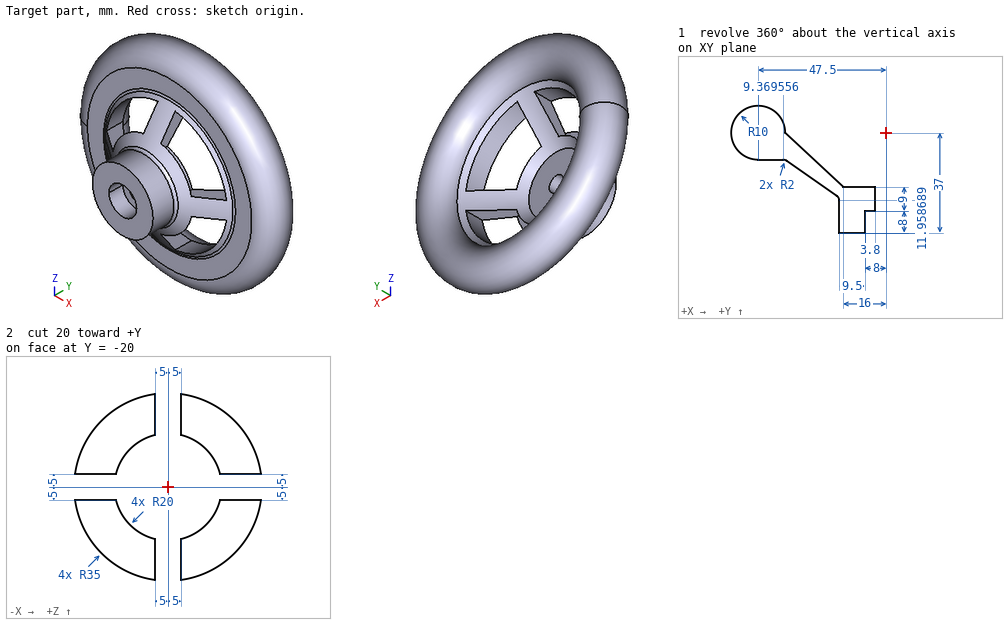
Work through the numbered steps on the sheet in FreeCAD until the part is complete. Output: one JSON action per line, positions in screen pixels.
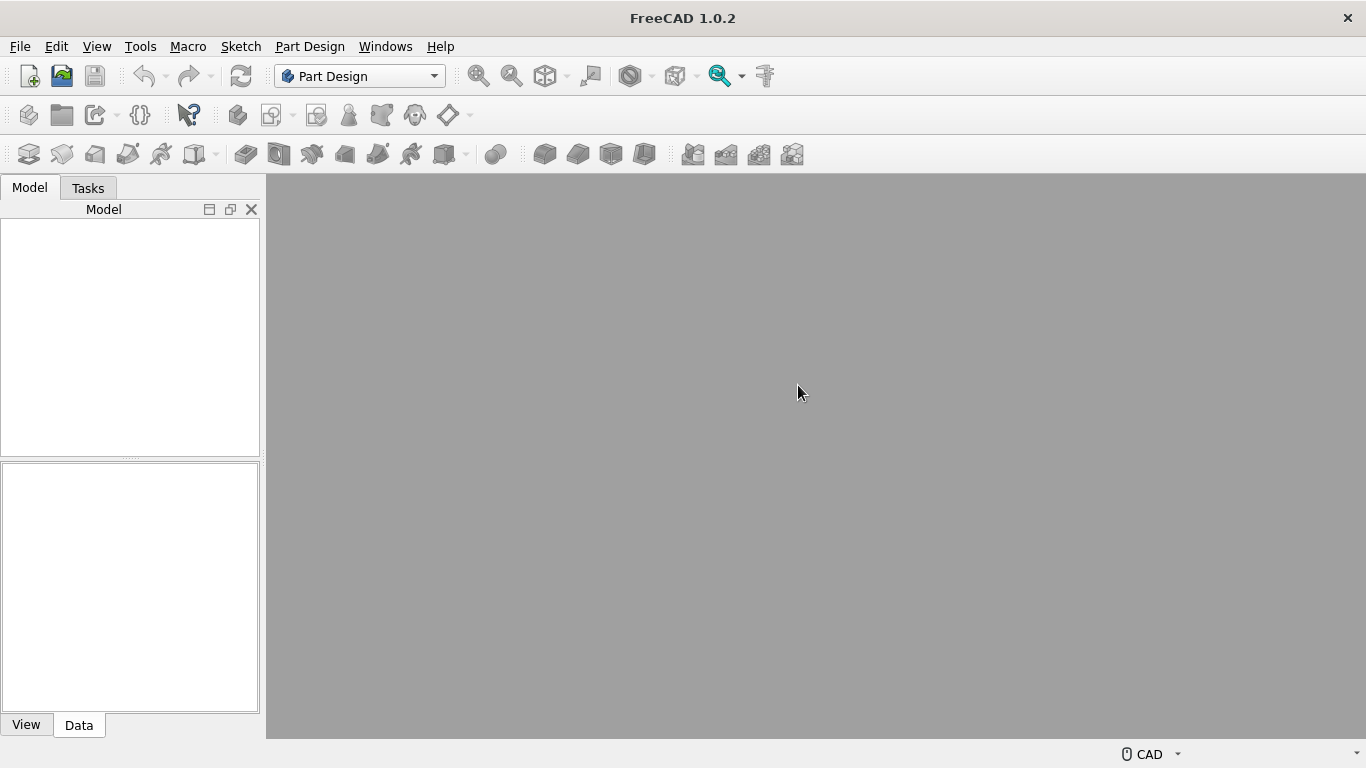
{"action": "left_click", "coordinate": [29, 76]}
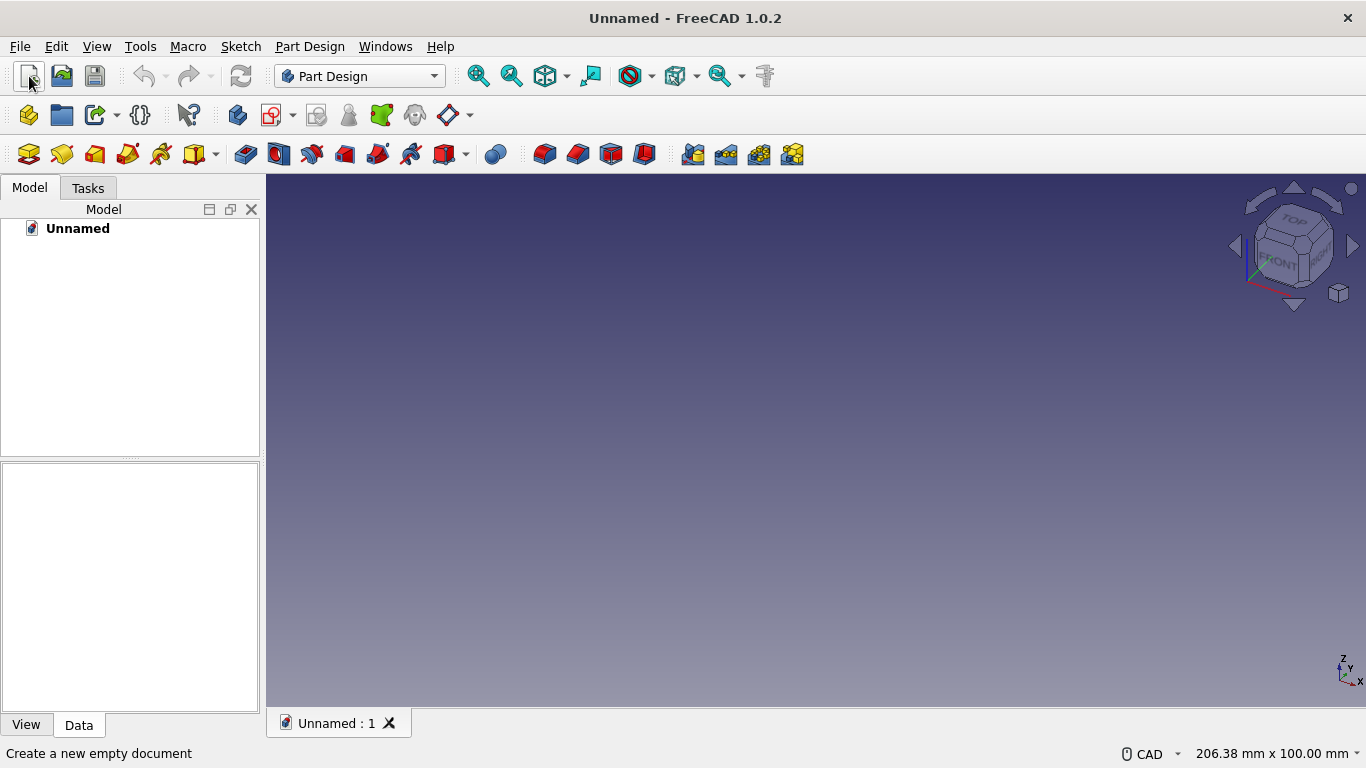
{"action": "left_click", "coordinate": [270, 116]}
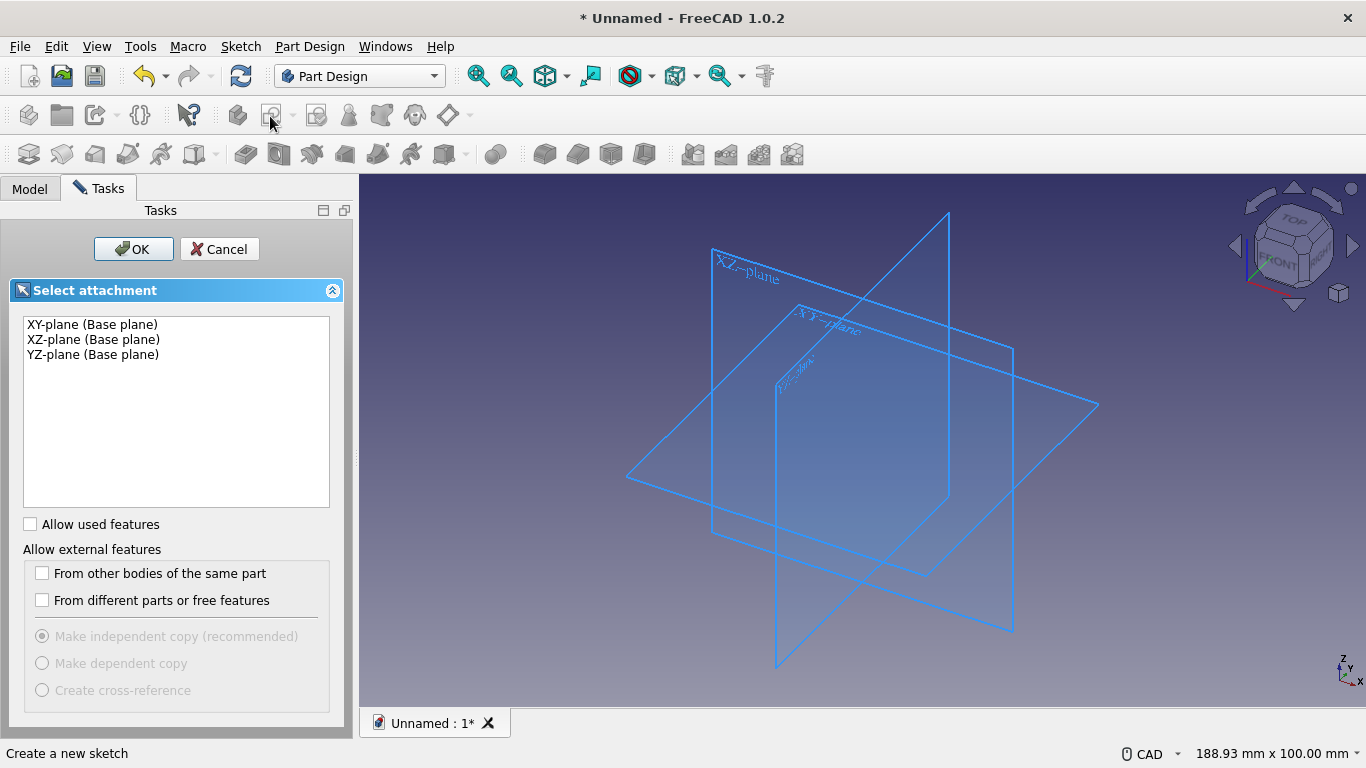
{"action": "left_click", "coordinate": [84, 324]}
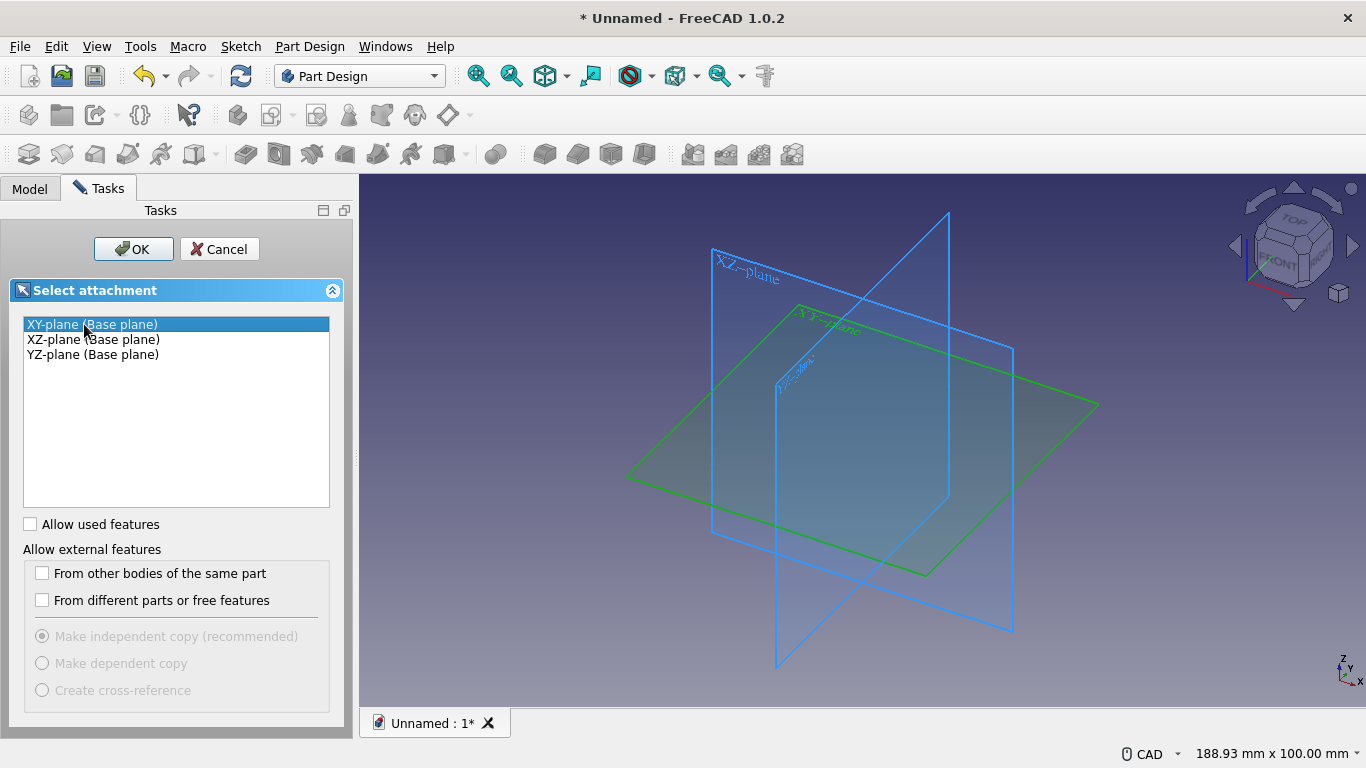
{"action": "left_click", "coordinate": [134, 249]}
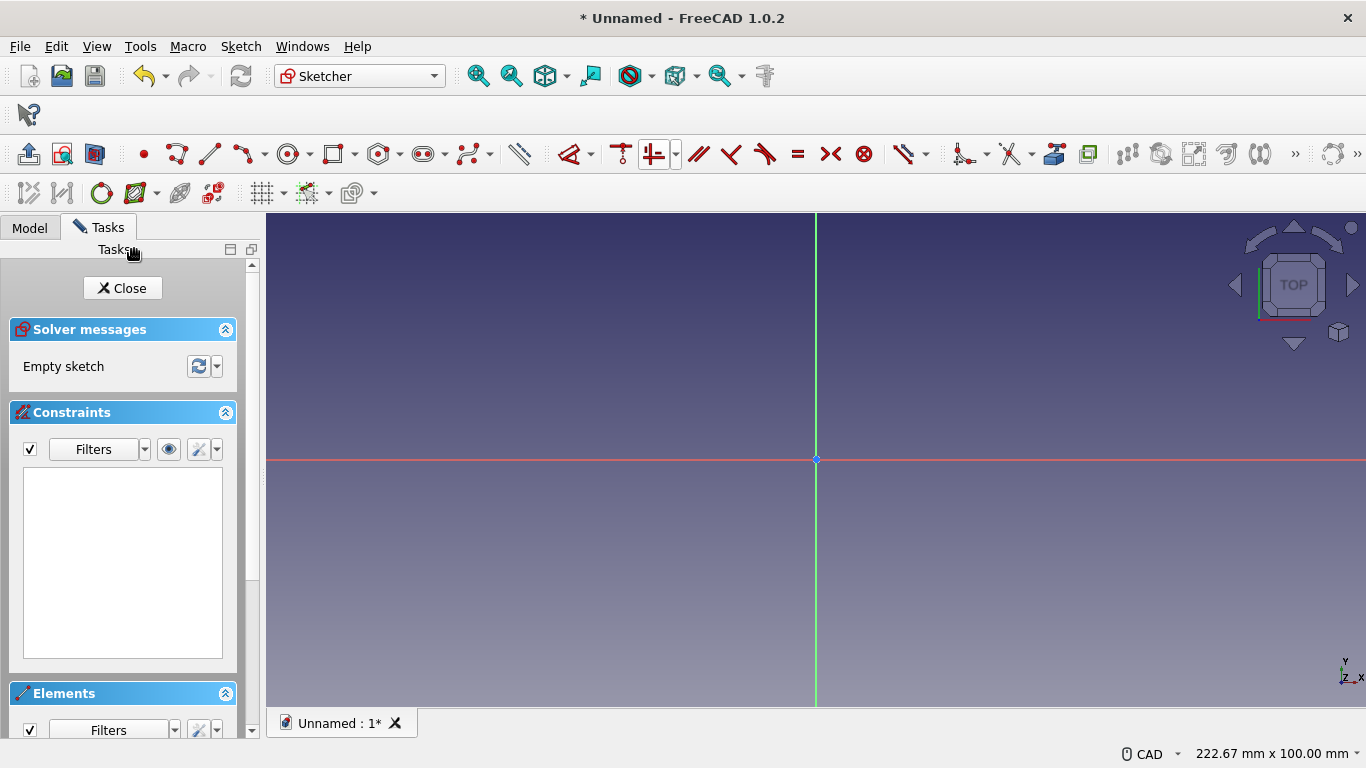
{"action": "scroll", "coordinate": [546, 679], "scroll_direction": "up", "scroll_amount": 2}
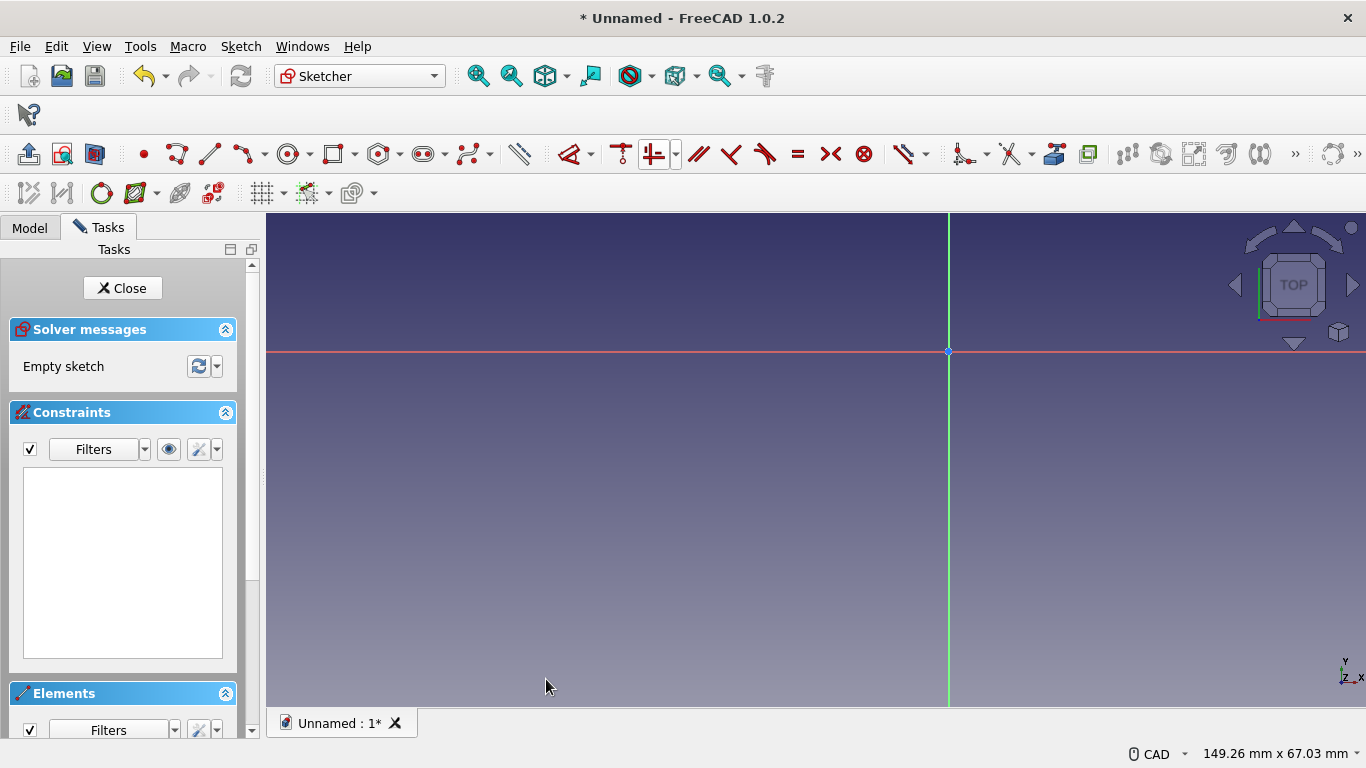
{"action": "key", "text": "g l"}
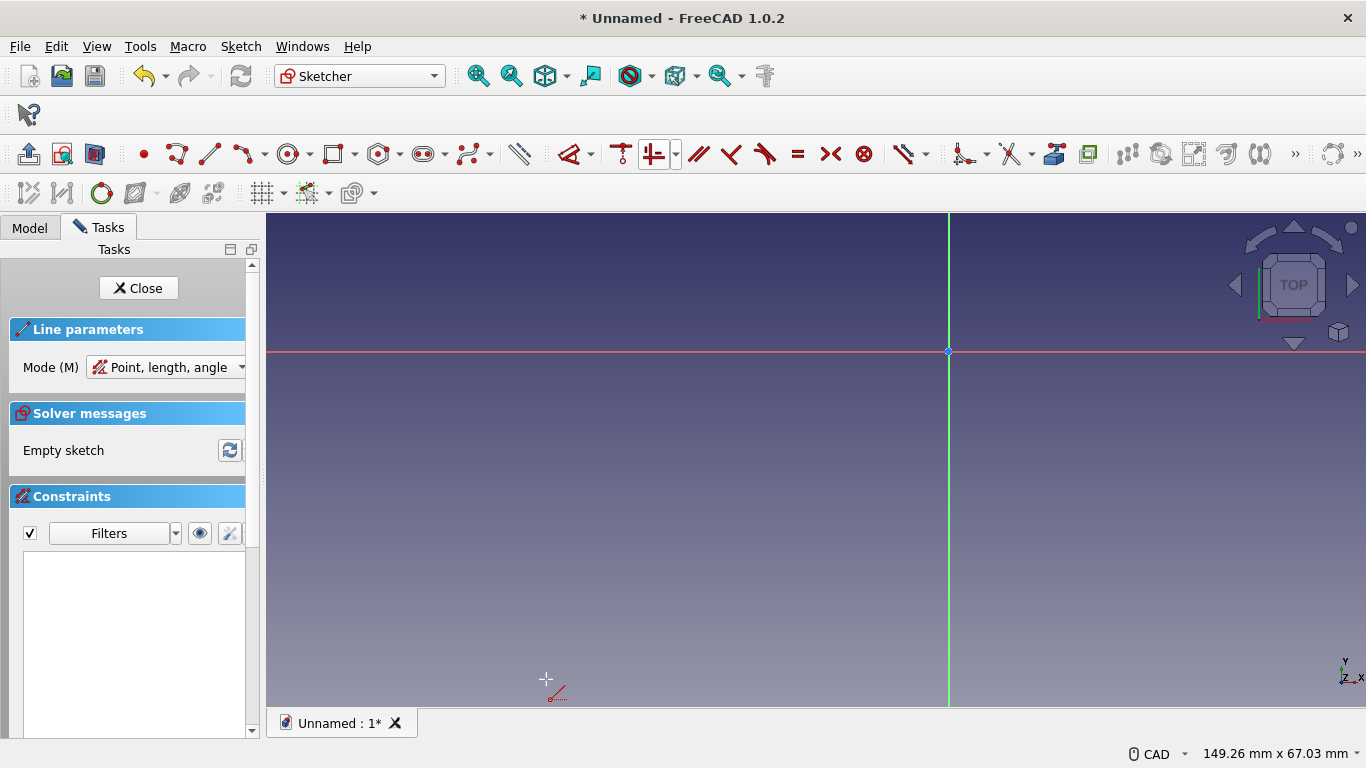
{"action": "left_click", "coordinate": [599, 426]}
{"action": "left_click", "coordinate": [668, 426]}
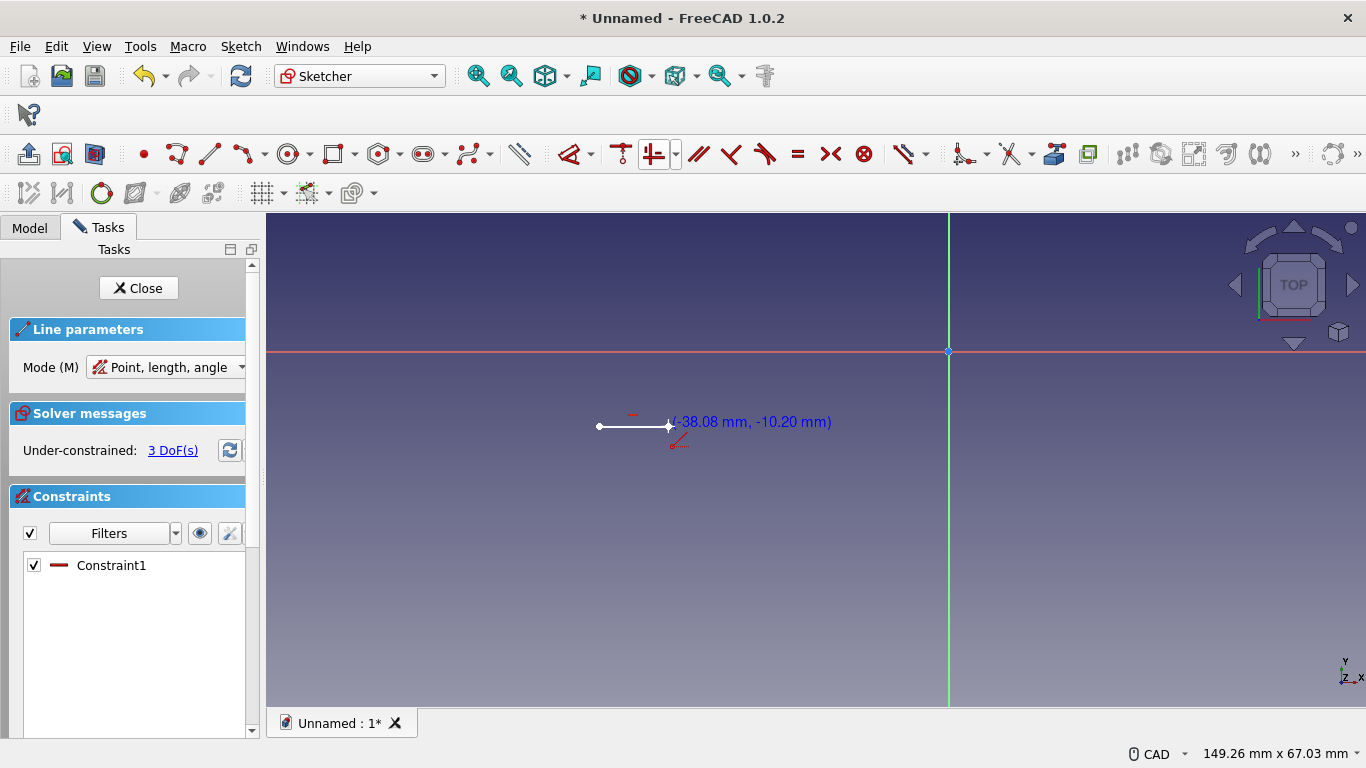
{"action": "scroll", "coordinate": [676, 428], "scroll_direction": "up", "scroll_amount": 3}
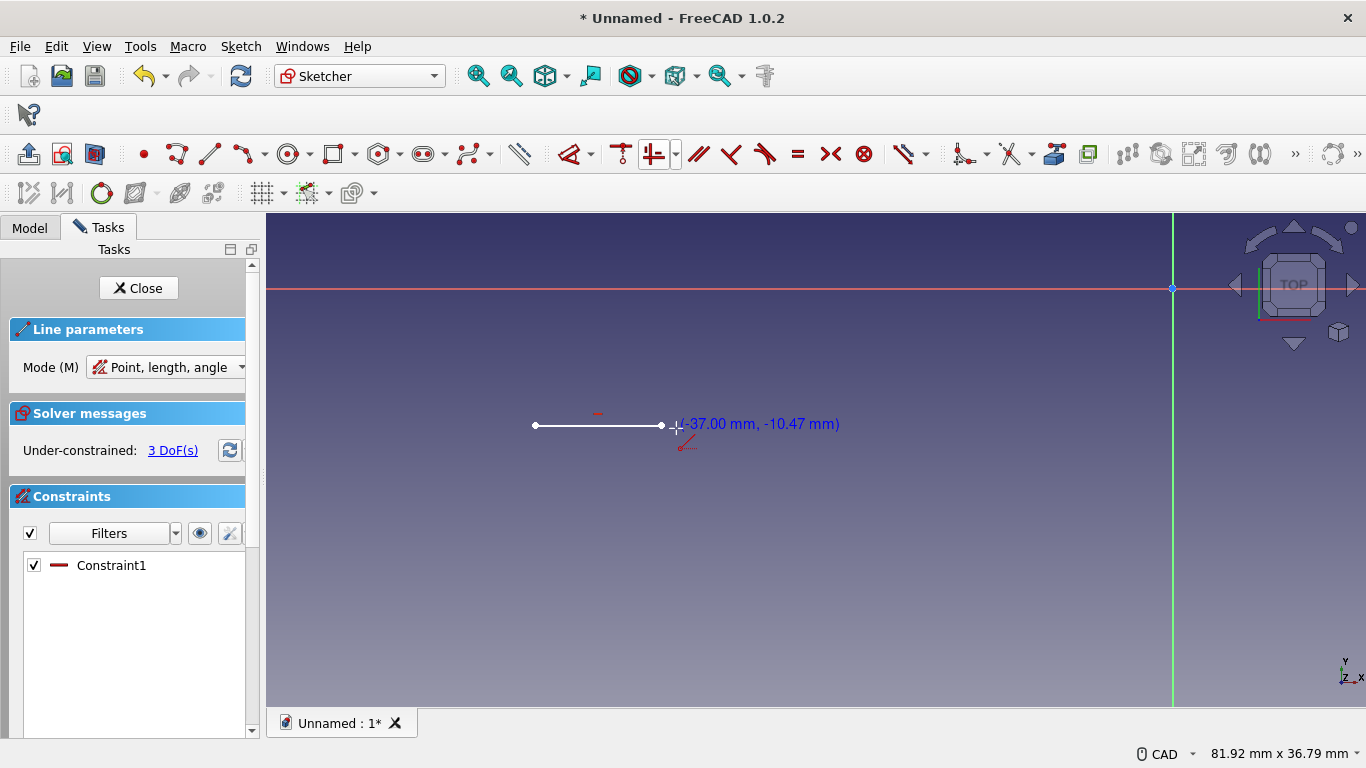
{"action": "left_click", "coordinate": [676, 428]}
{"action": "left_click", "coordinate": [926, 603]}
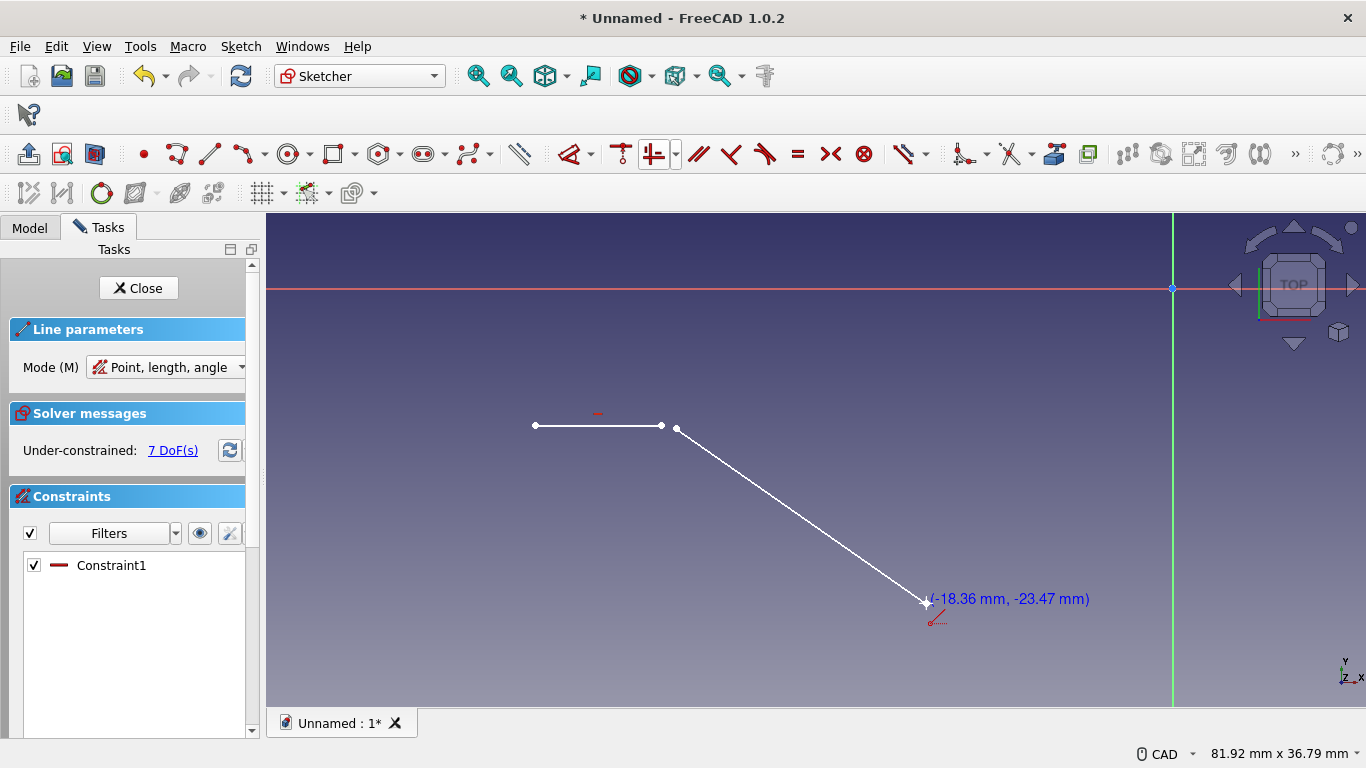
{"action": "key", "text": "g m"}